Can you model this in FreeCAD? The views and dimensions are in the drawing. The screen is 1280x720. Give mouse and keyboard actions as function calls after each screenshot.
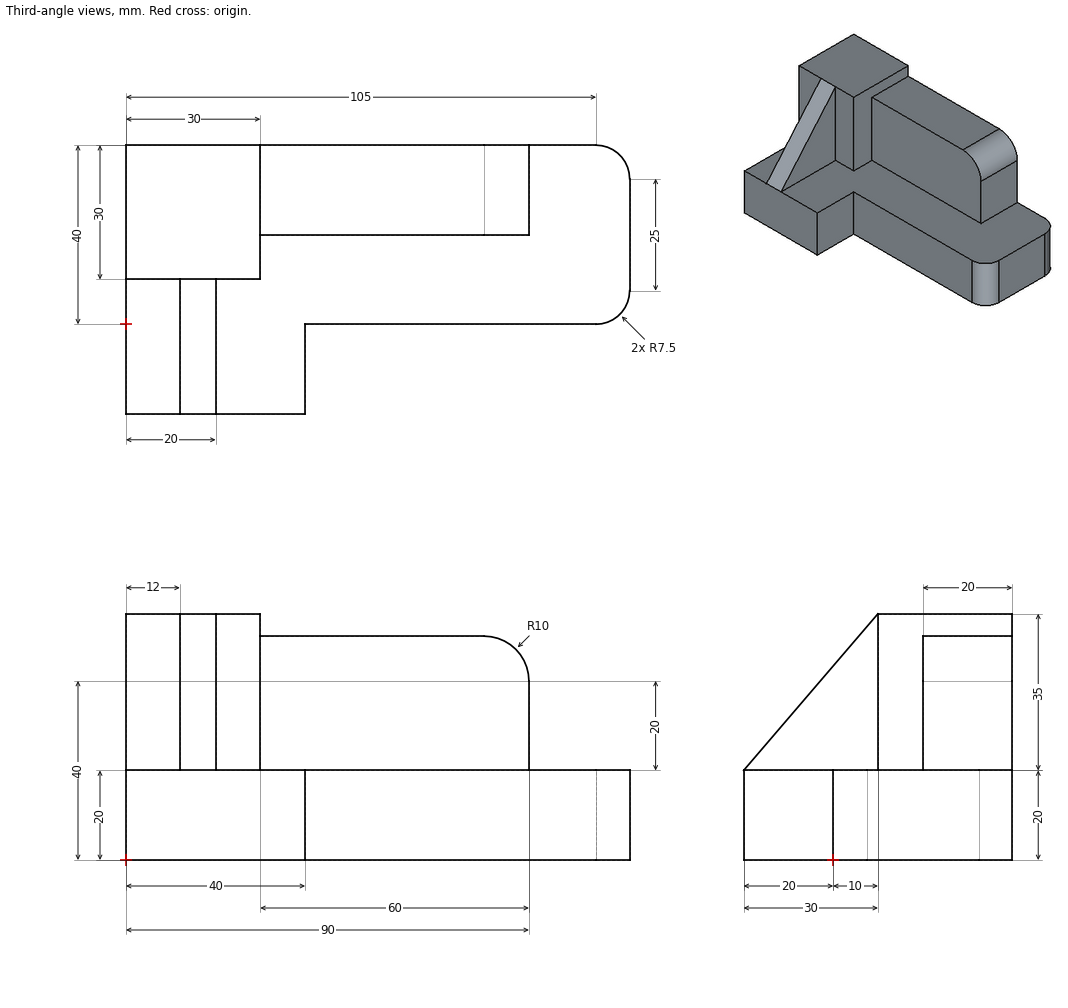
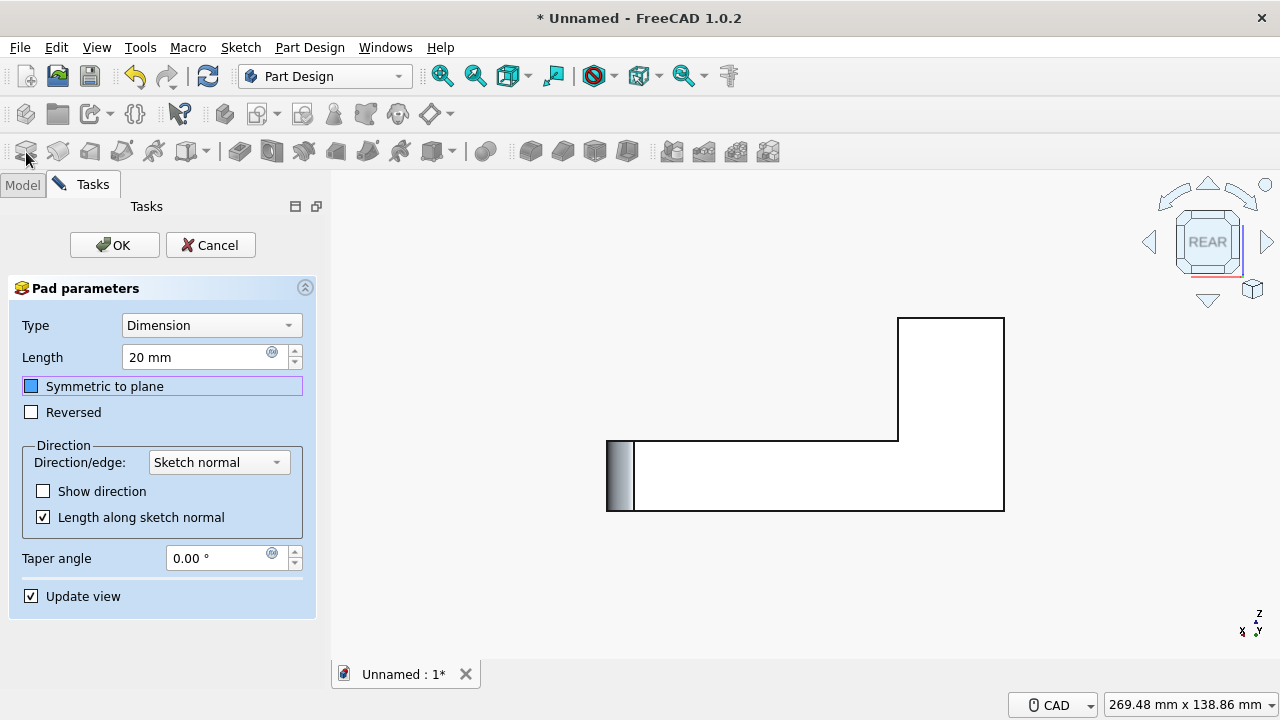
click(30, 412)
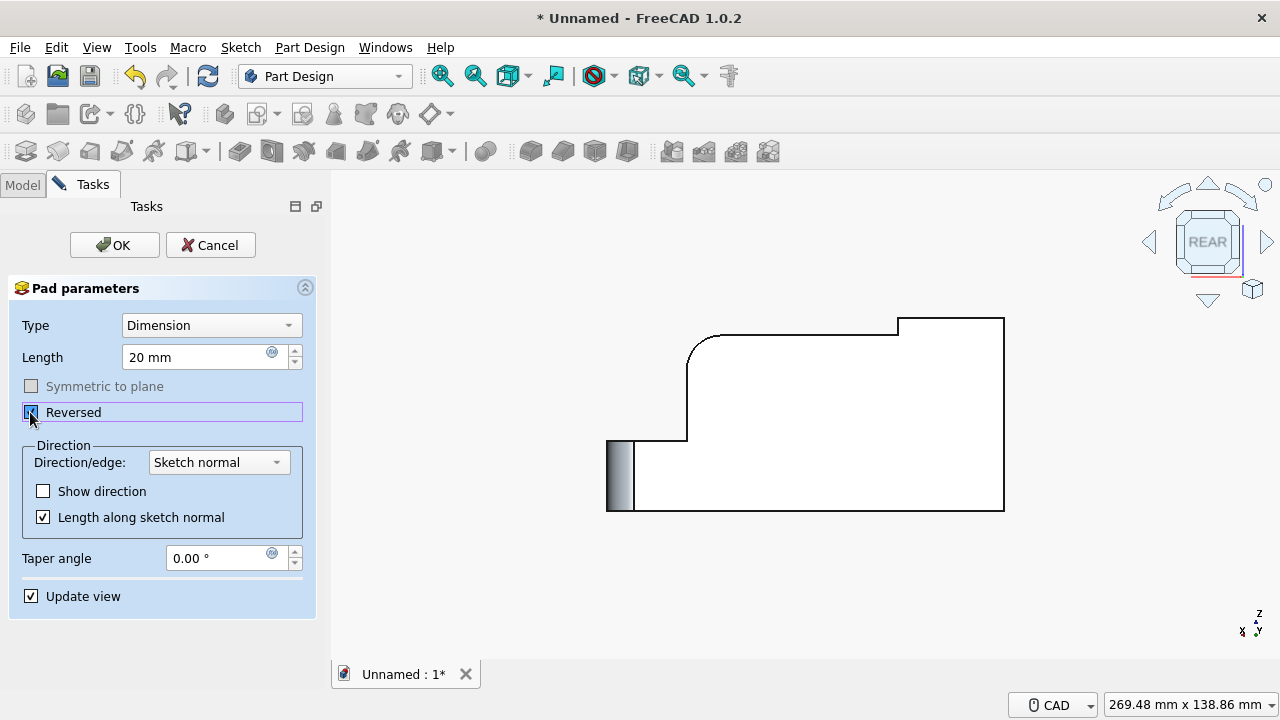
click(115, 245)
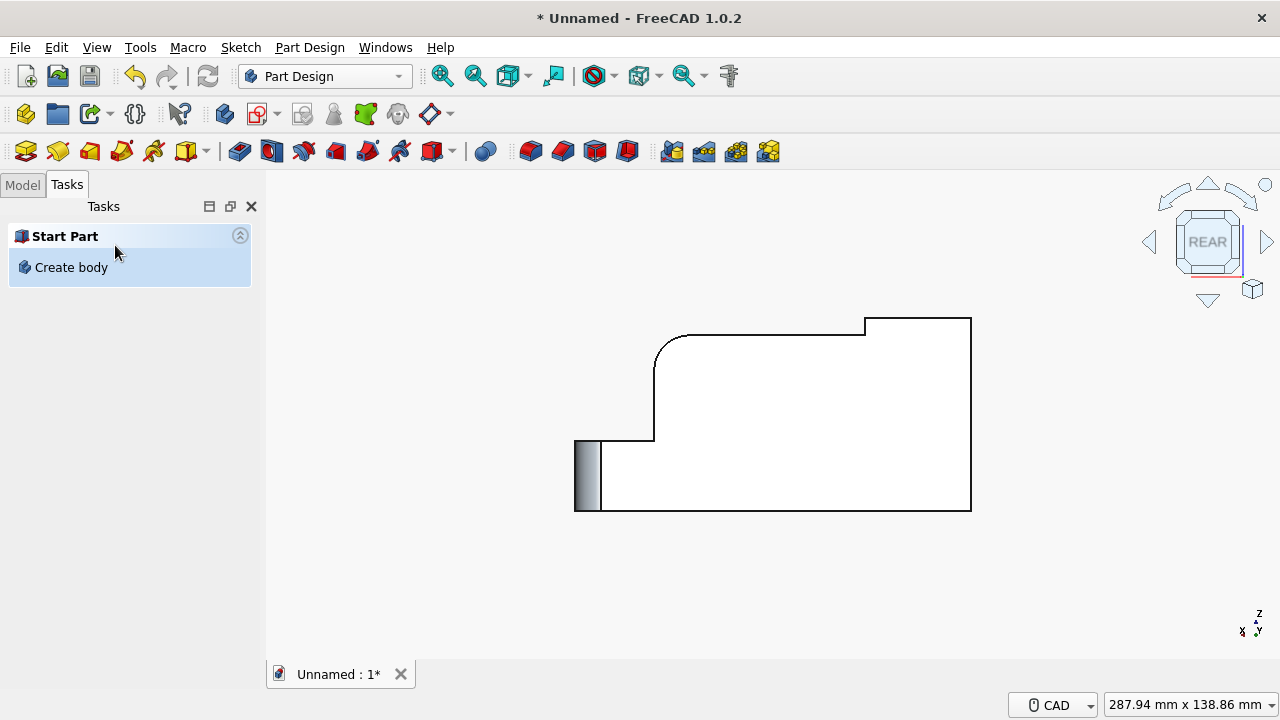
key(v)
key(f)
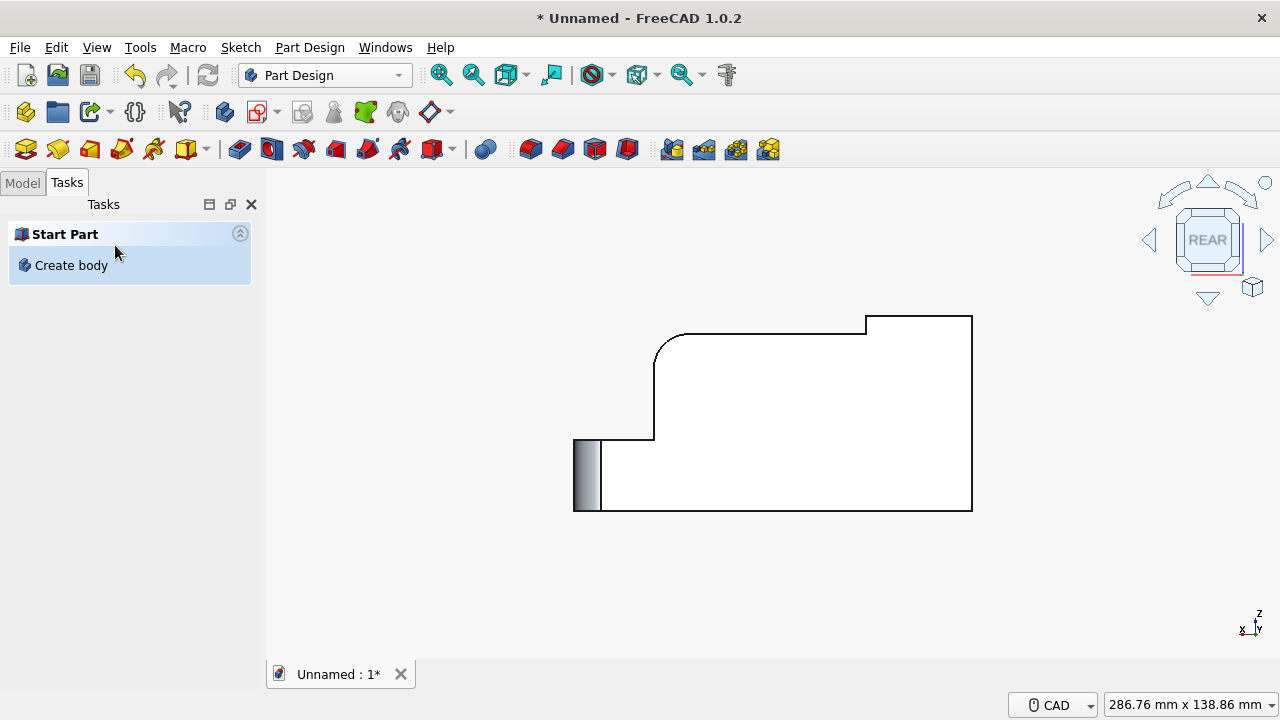
click(258, 112)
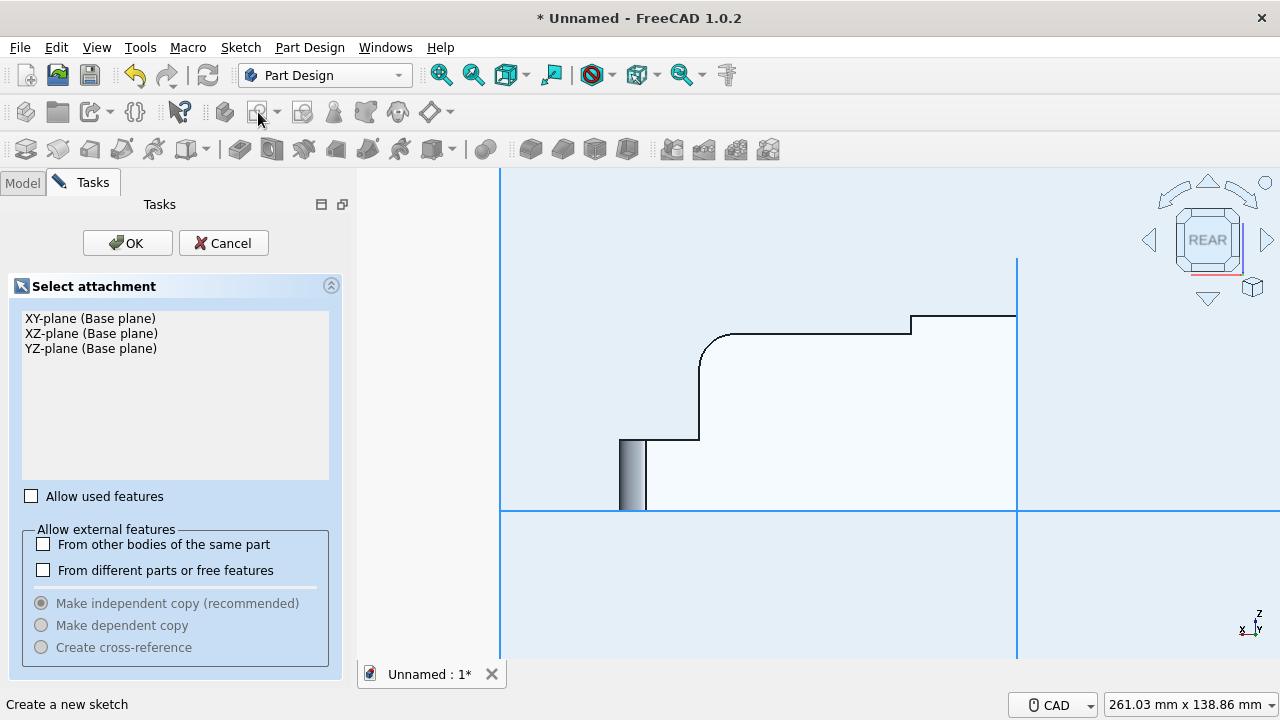
click(82, 348)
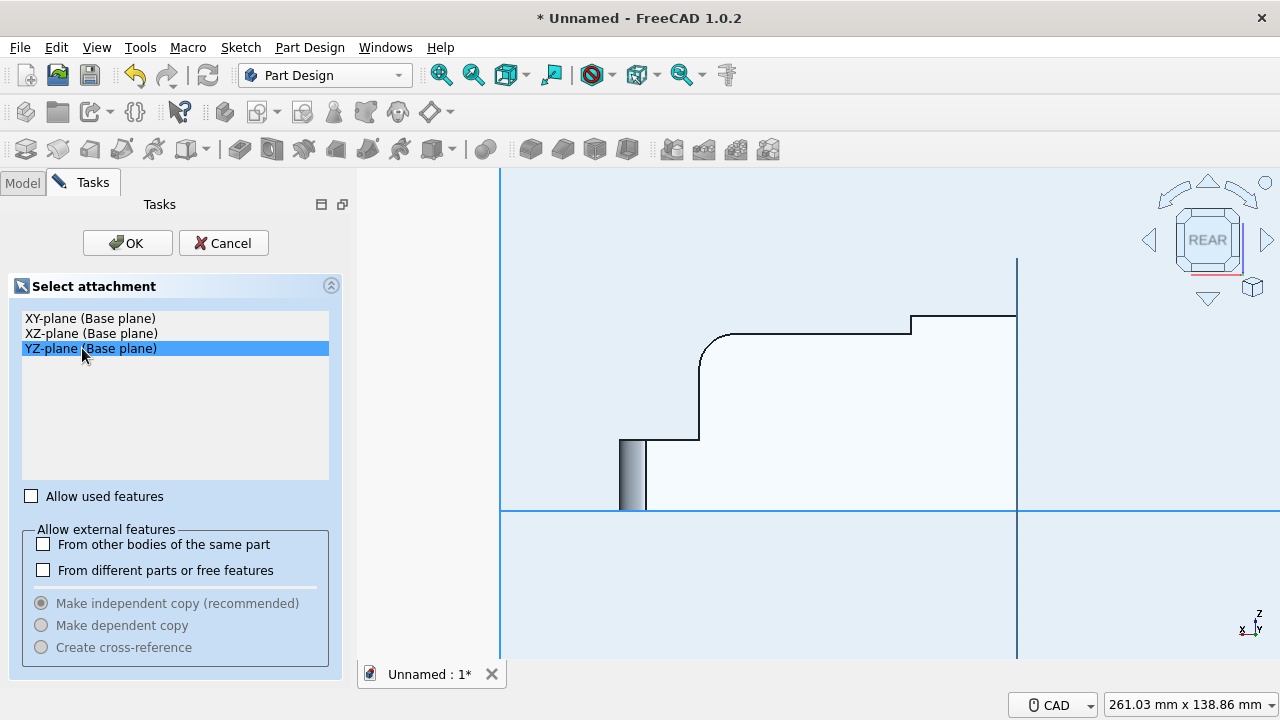
click(128, 243)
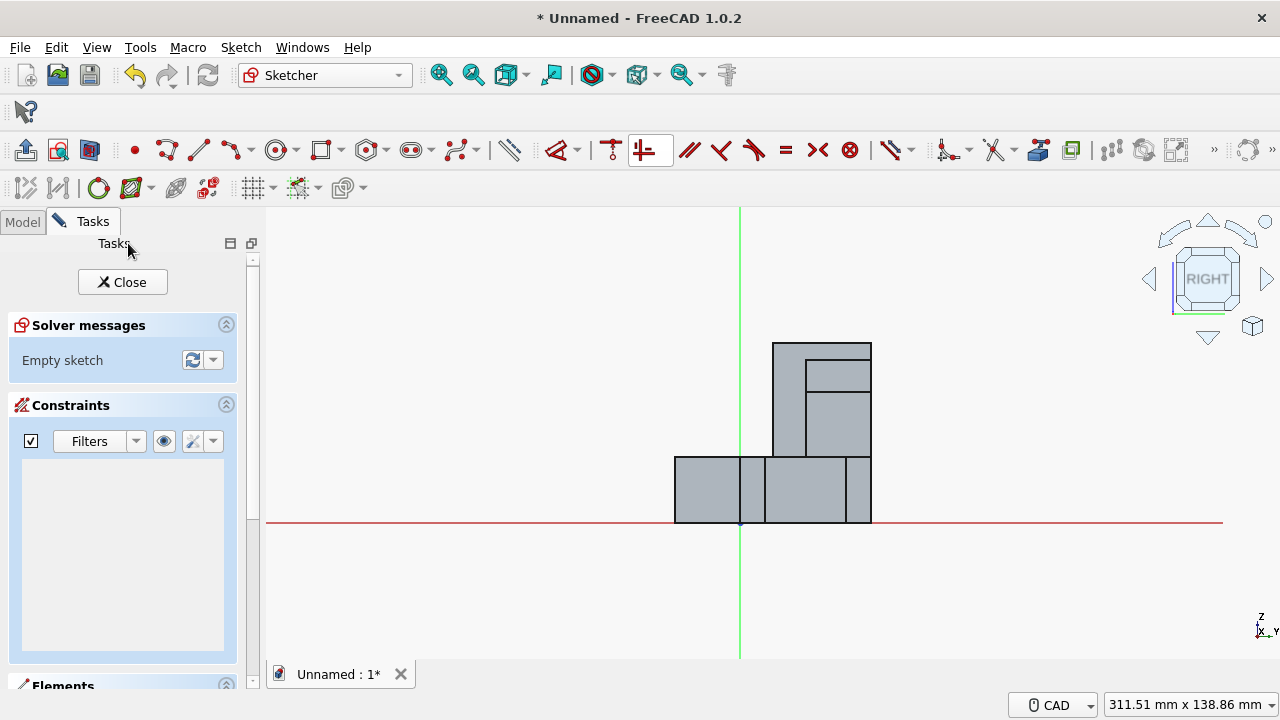
key(q)
key(s)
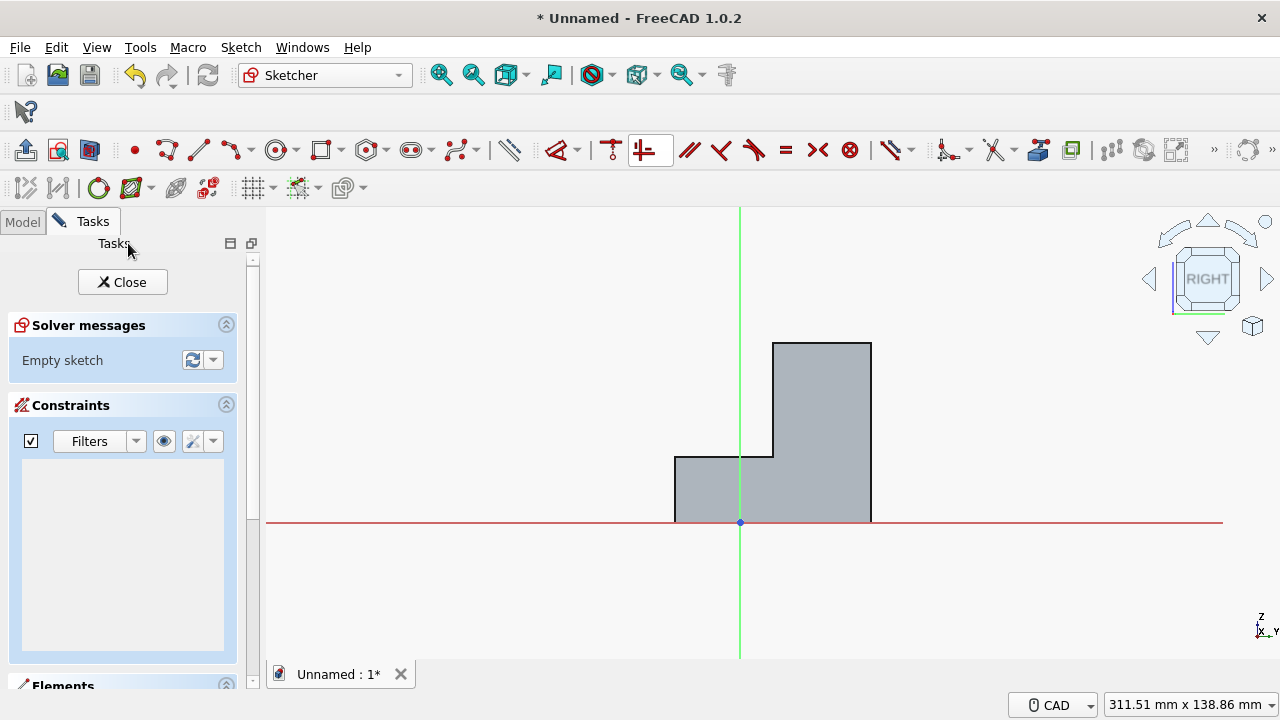
scroll(764, 433, up, 2)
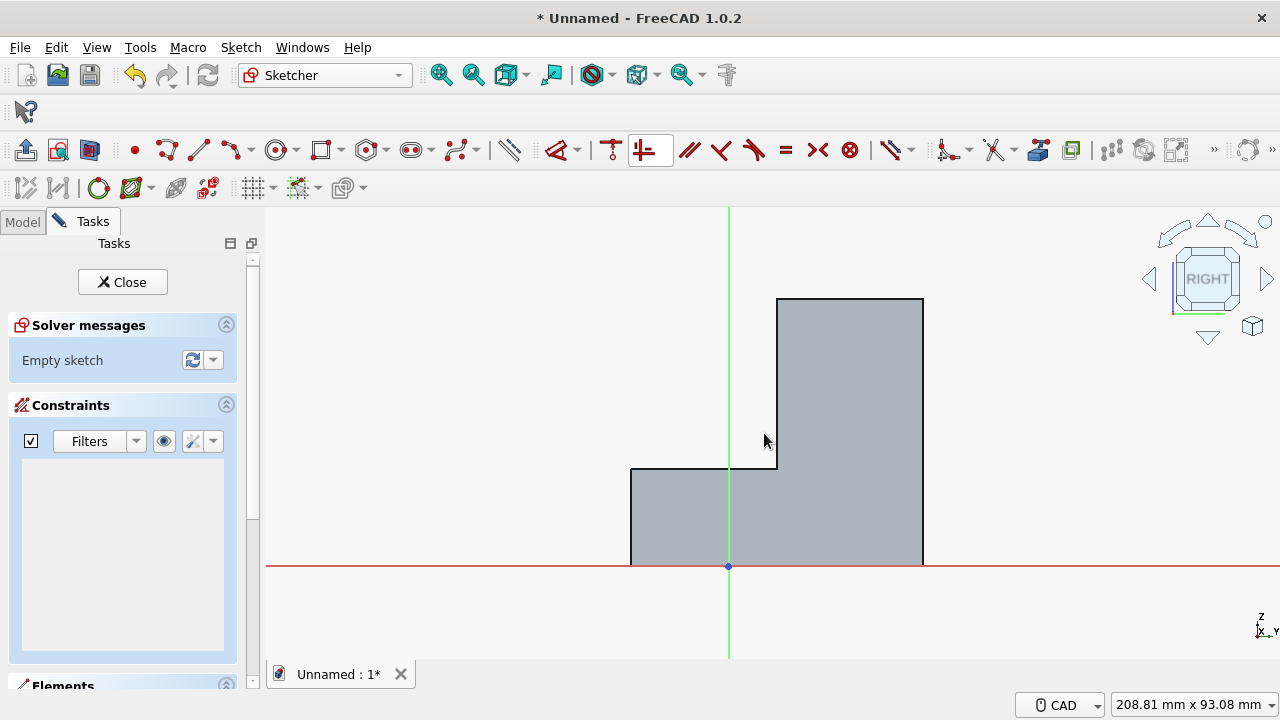
key(g)
key(m)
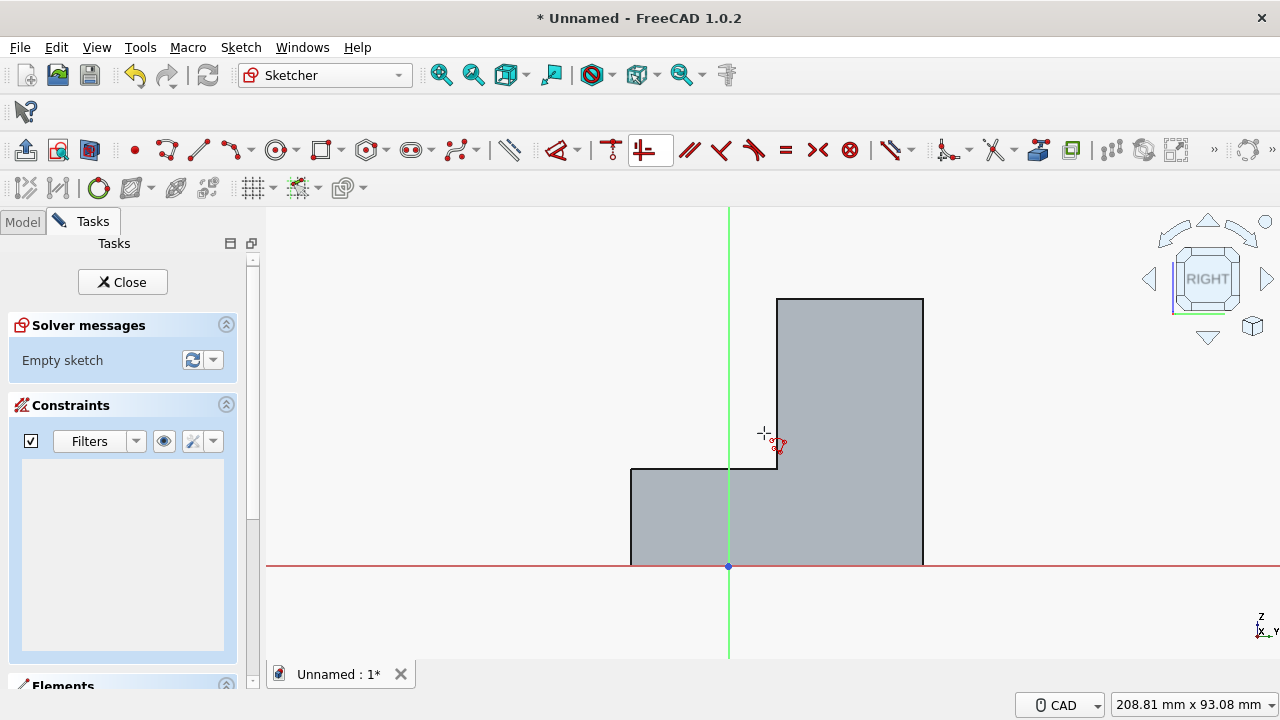
click(777, 469)
click(632, 469)
click(777, 299)
click(777, 470)
key(Escape)
key(Escape)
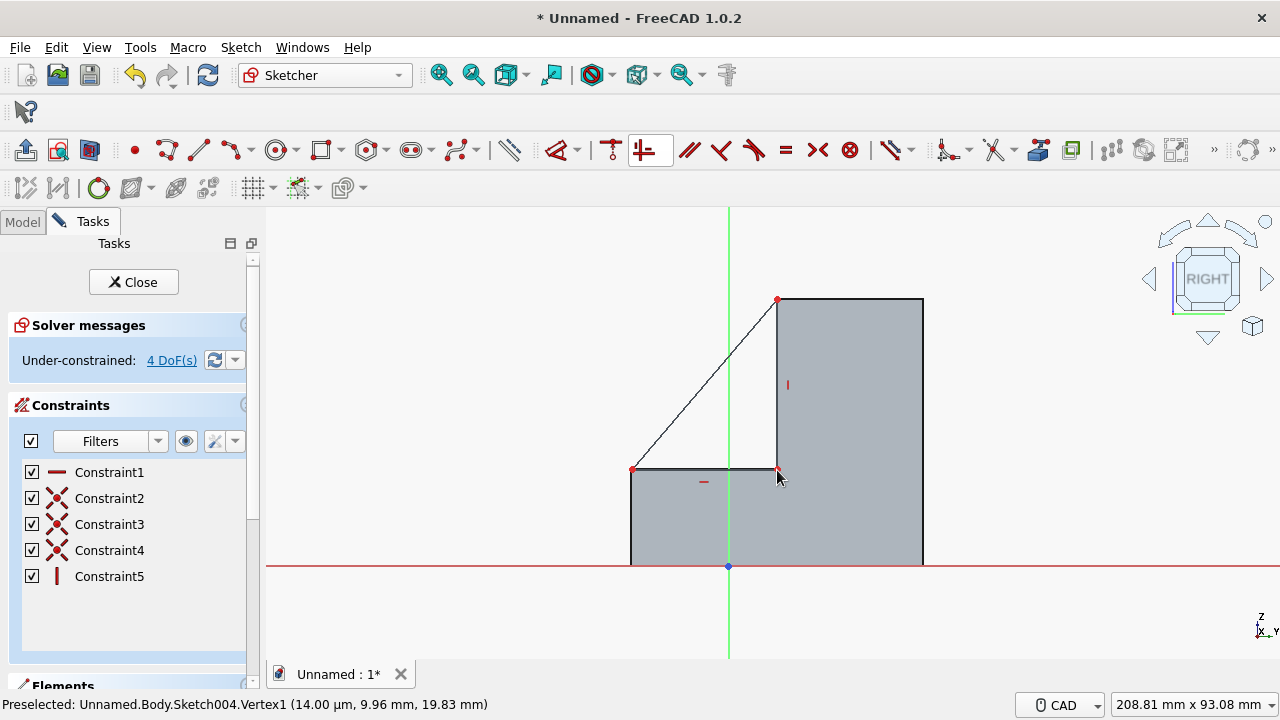
key(d)